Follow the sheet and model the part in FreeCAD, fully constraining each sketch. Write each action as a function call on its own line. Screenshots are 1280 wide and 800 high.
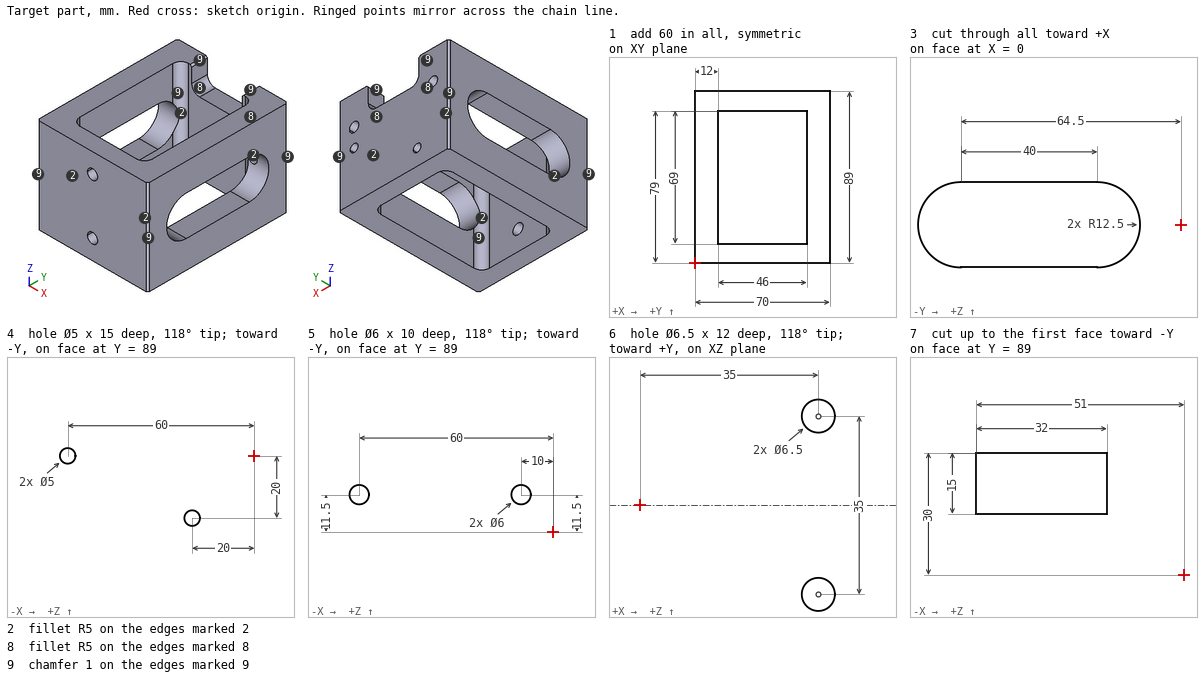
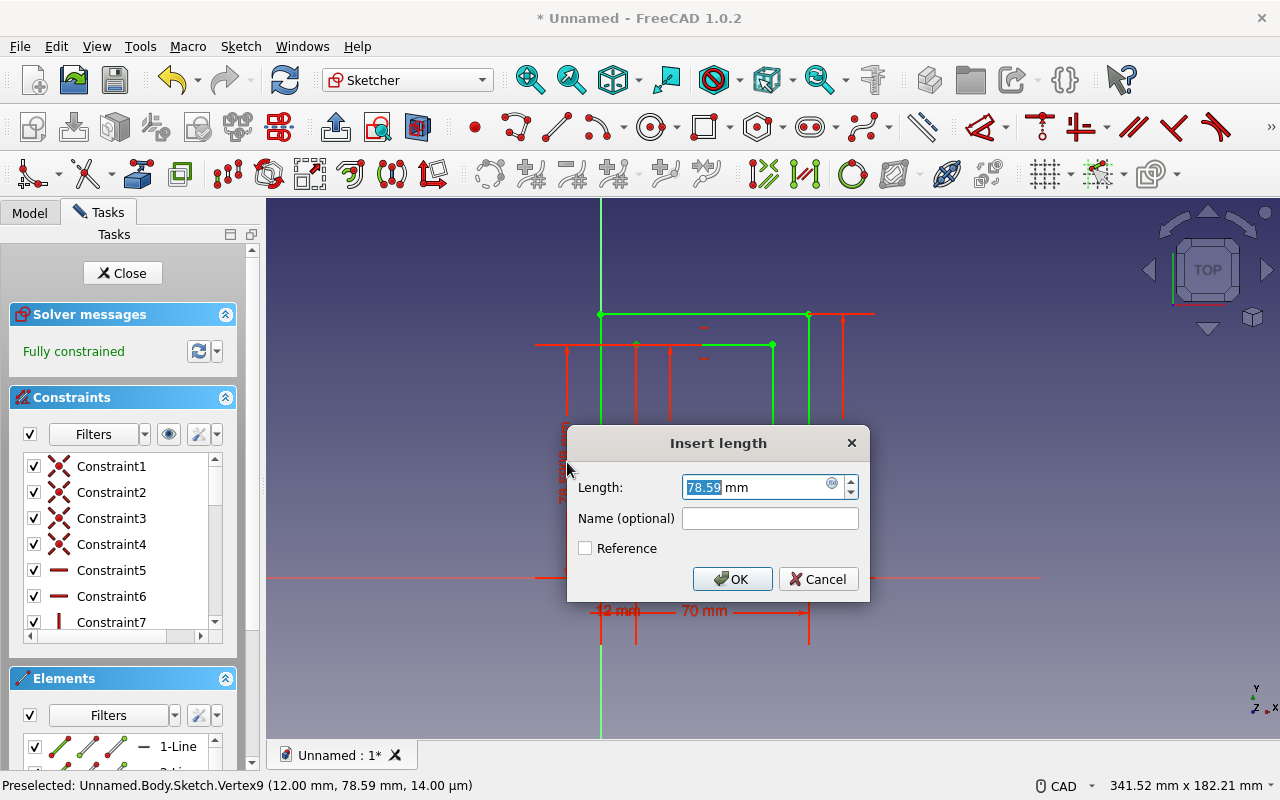
text(79)
key(Return)
key(Escape)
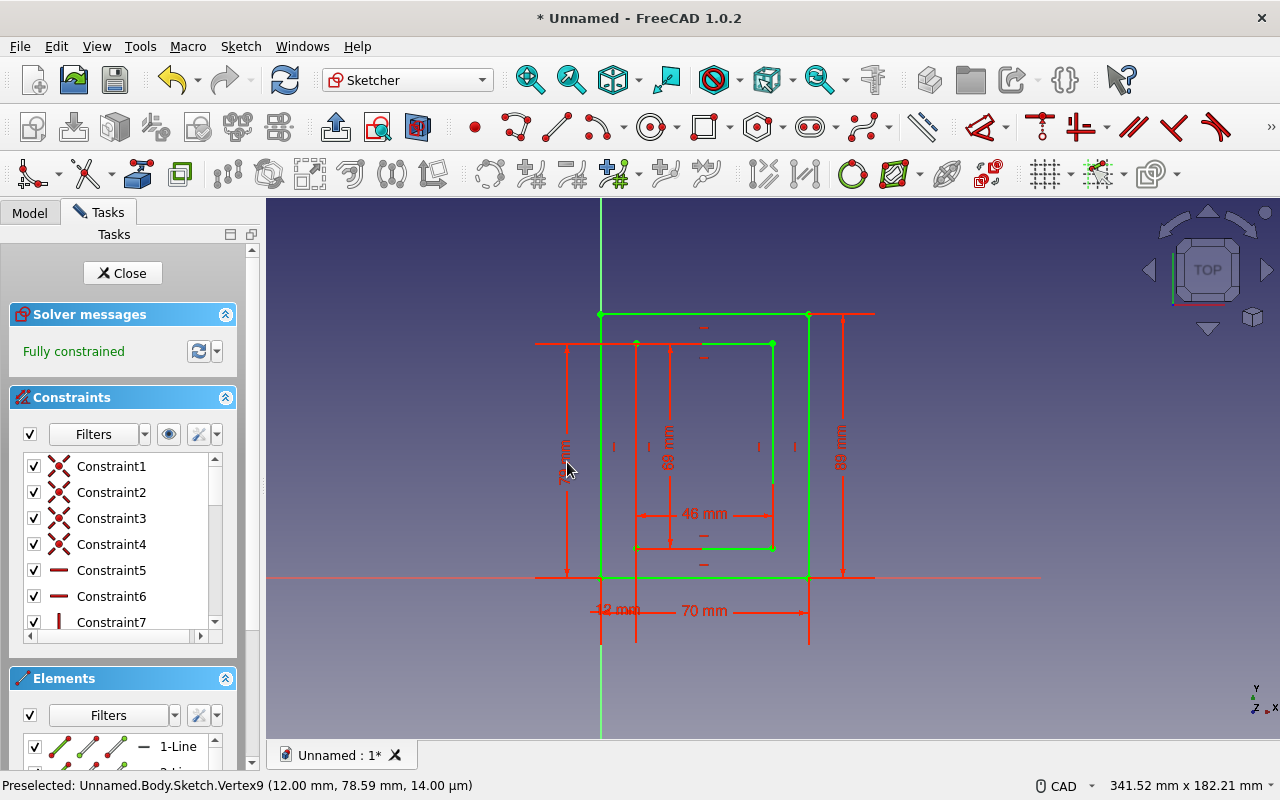
click(123, 273)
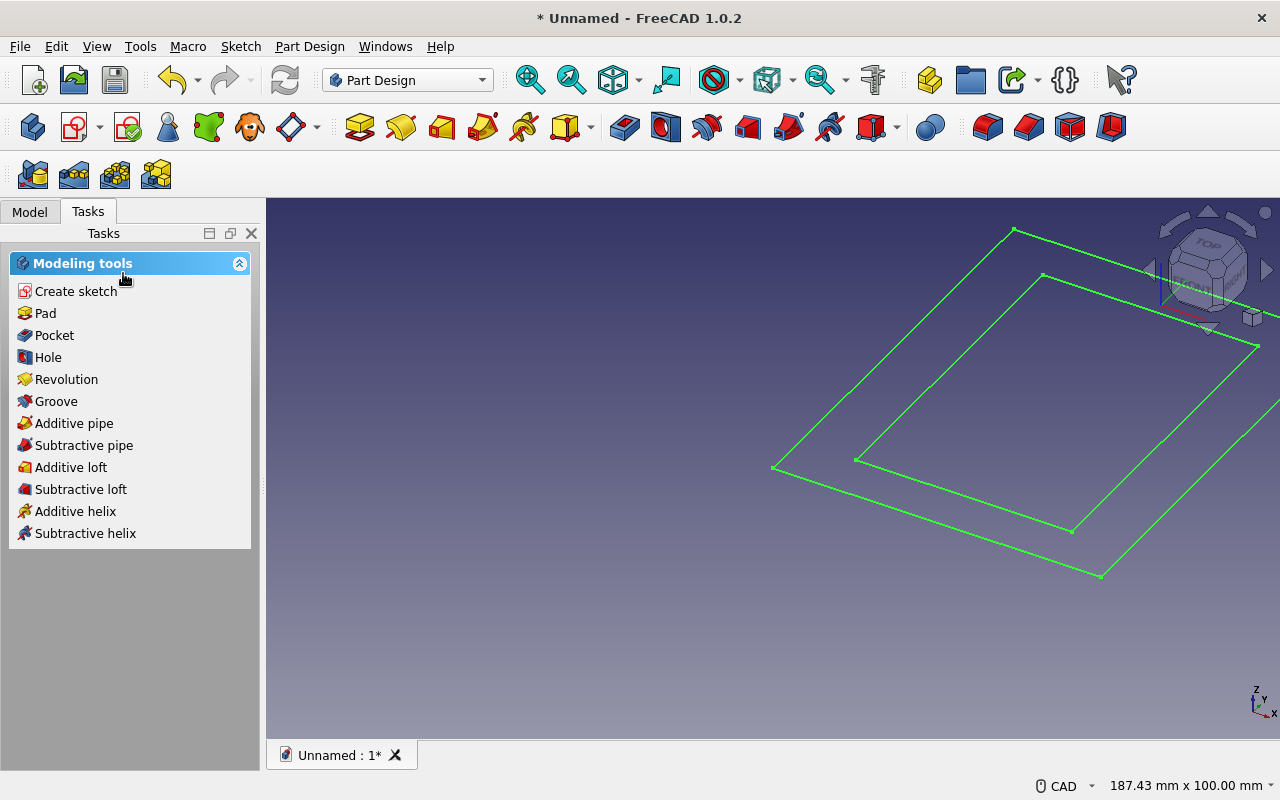
click(360, 128)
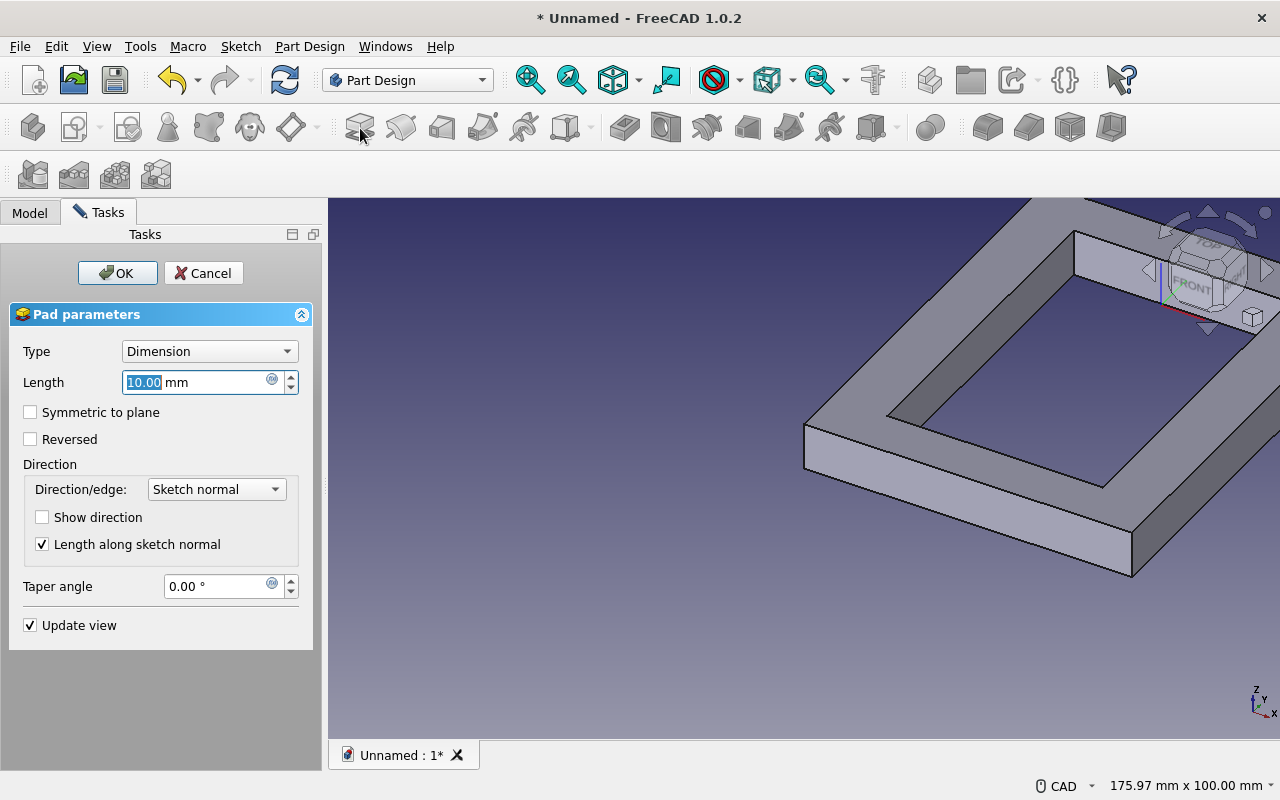
text(60)
key(Tab)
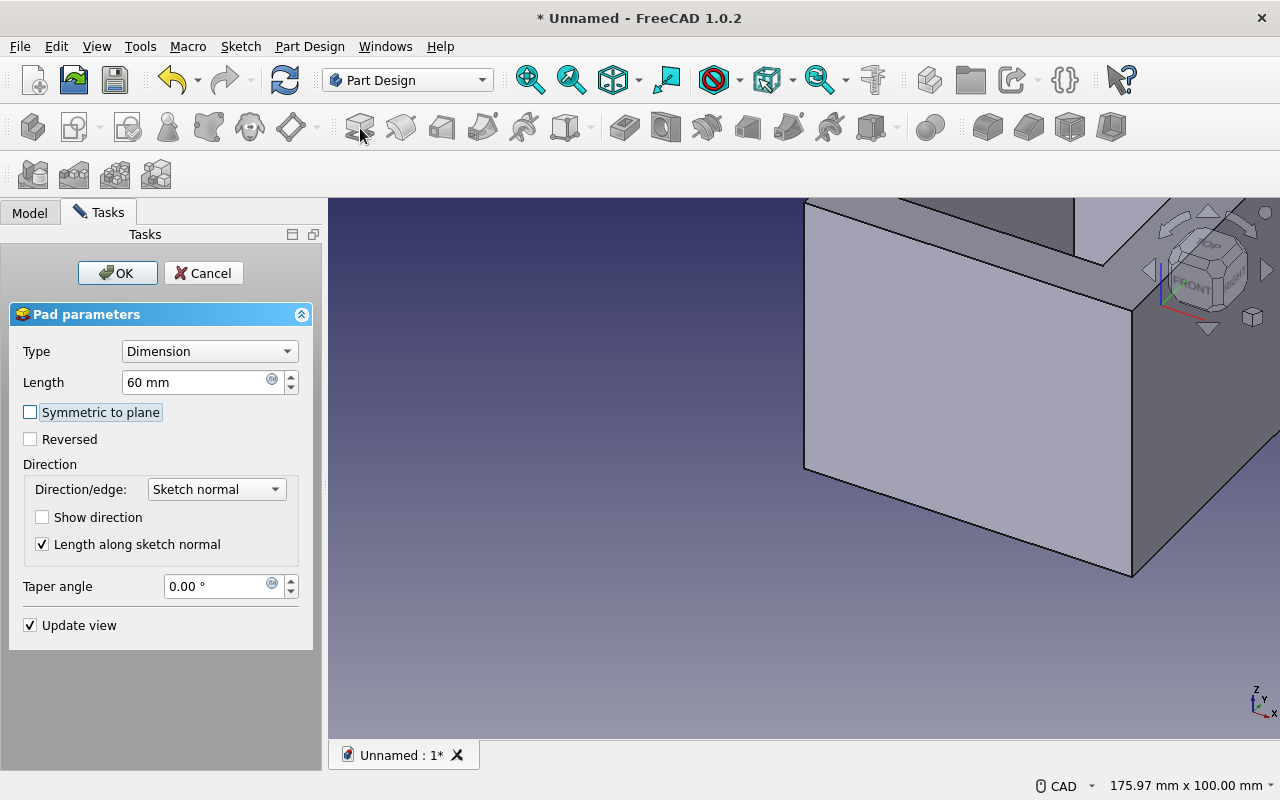
click(31, 412)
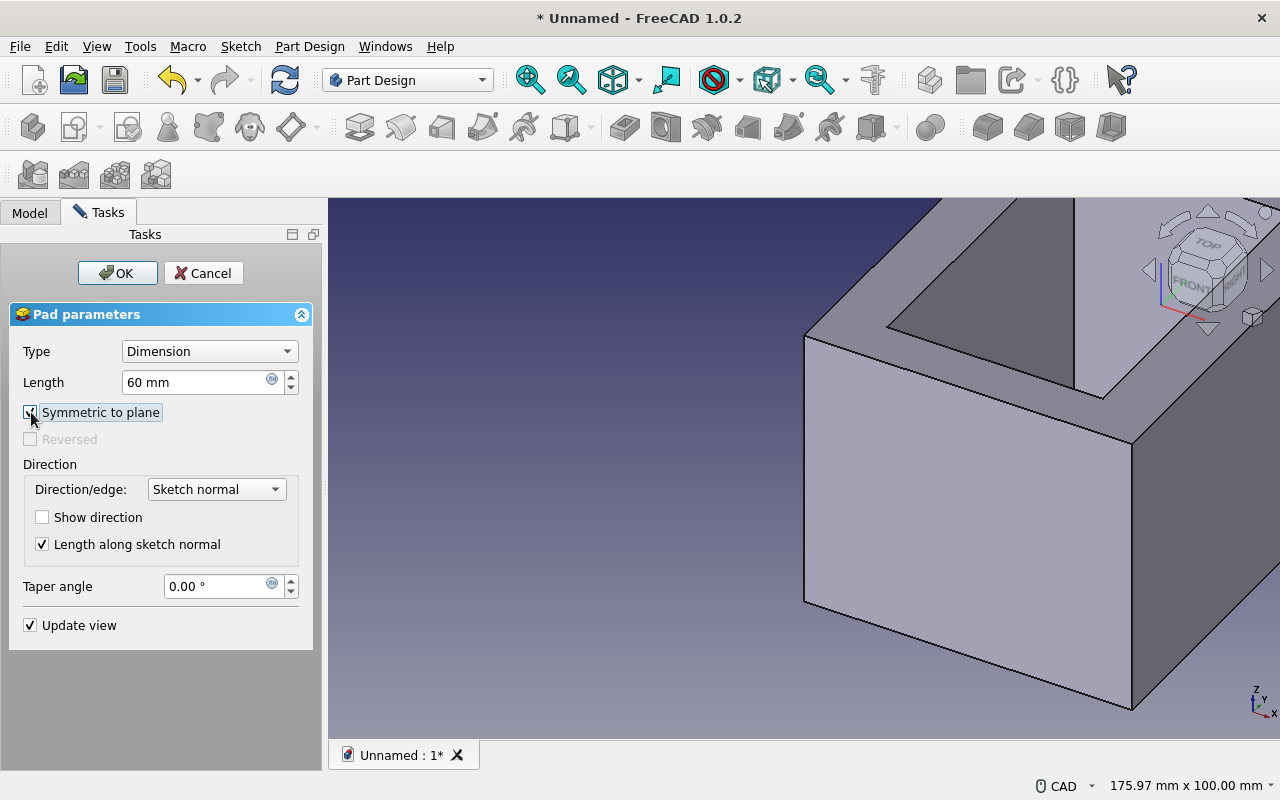
click(118, 273)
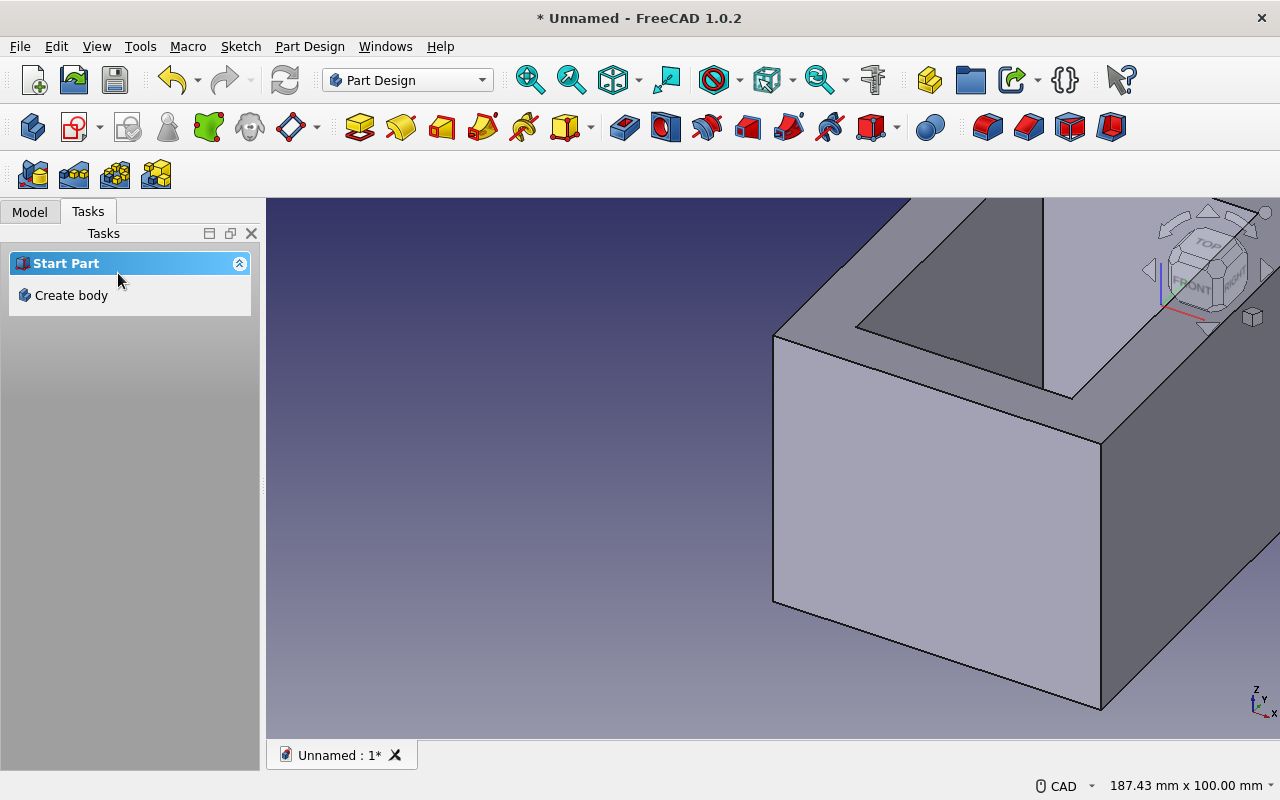
click(531, 80)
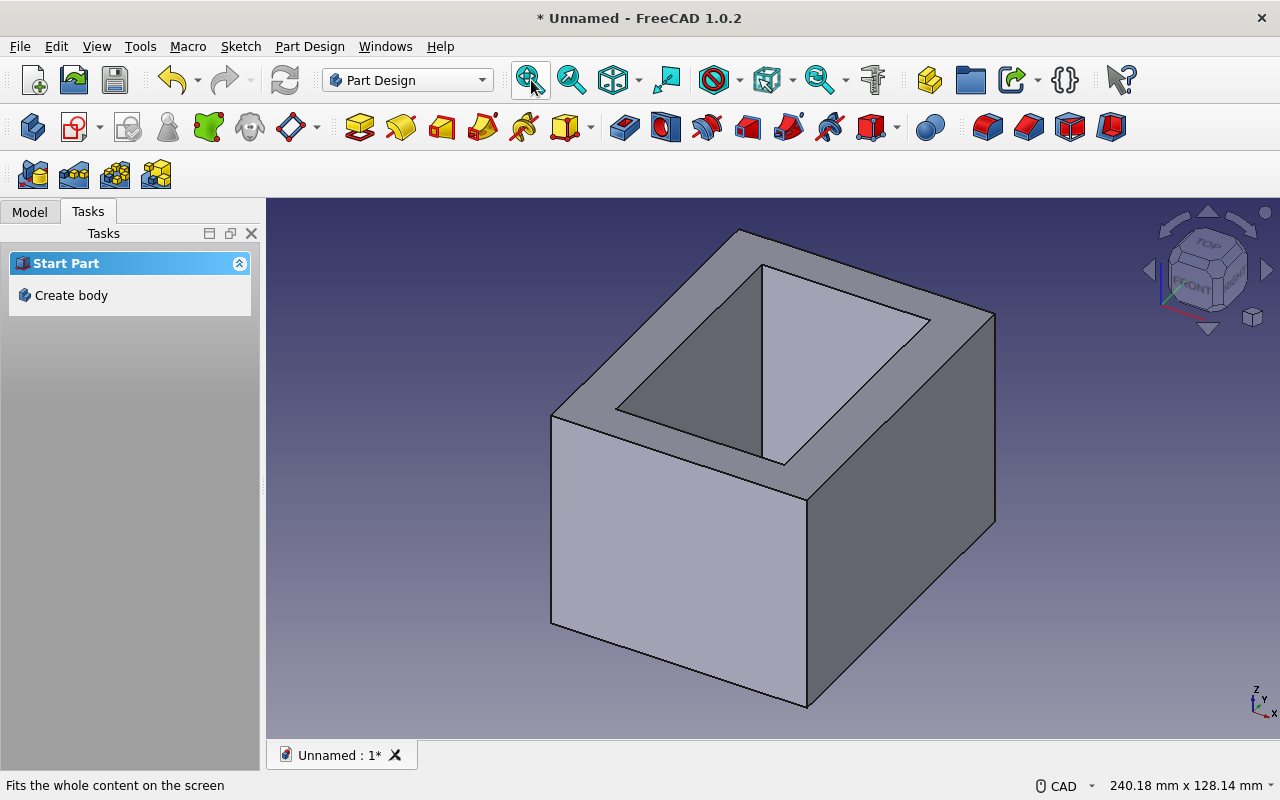
key(0)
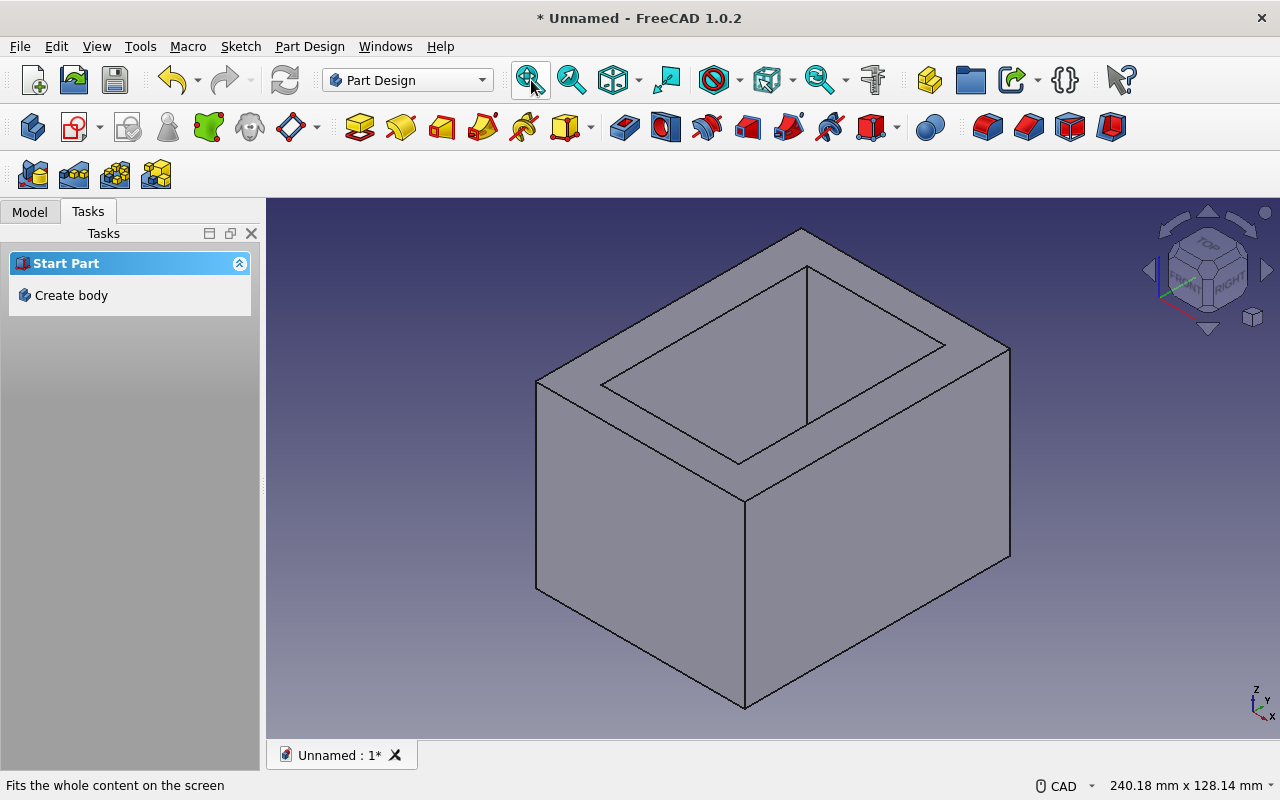
key(2)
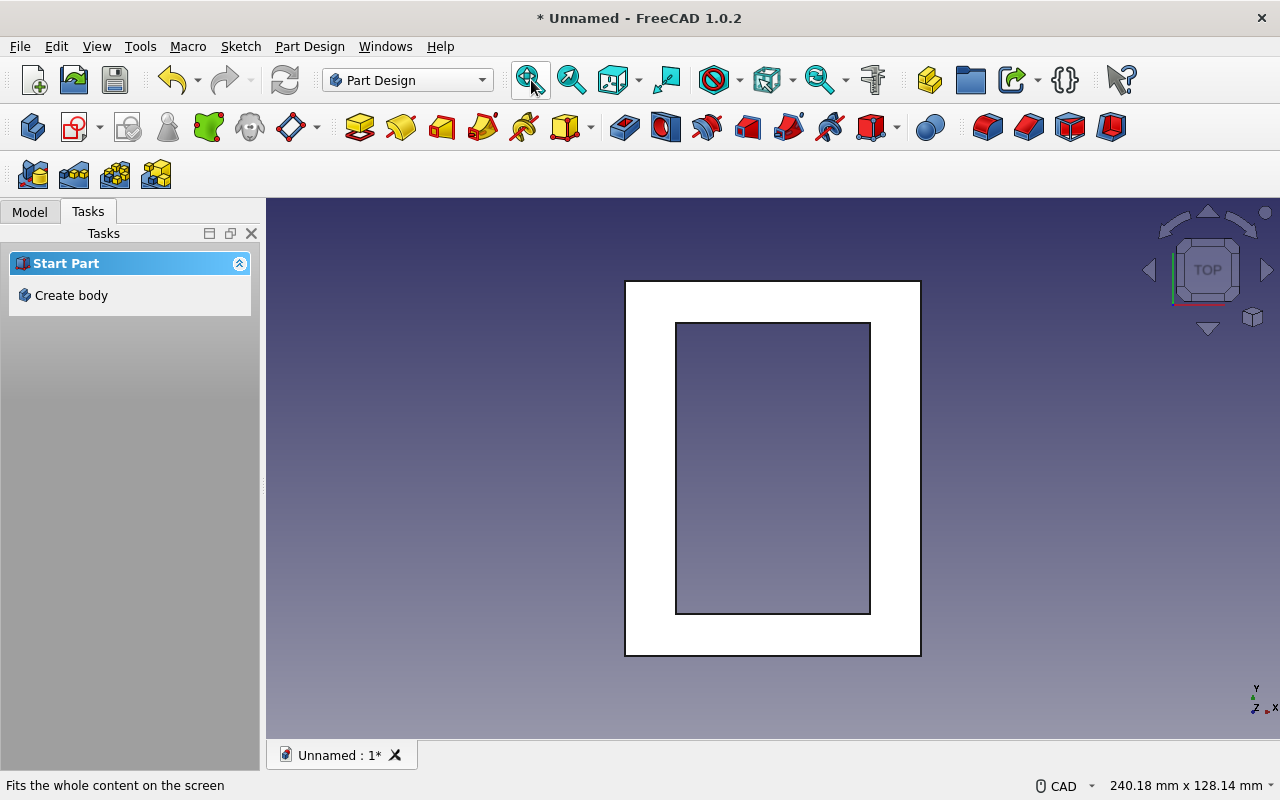
key(1)